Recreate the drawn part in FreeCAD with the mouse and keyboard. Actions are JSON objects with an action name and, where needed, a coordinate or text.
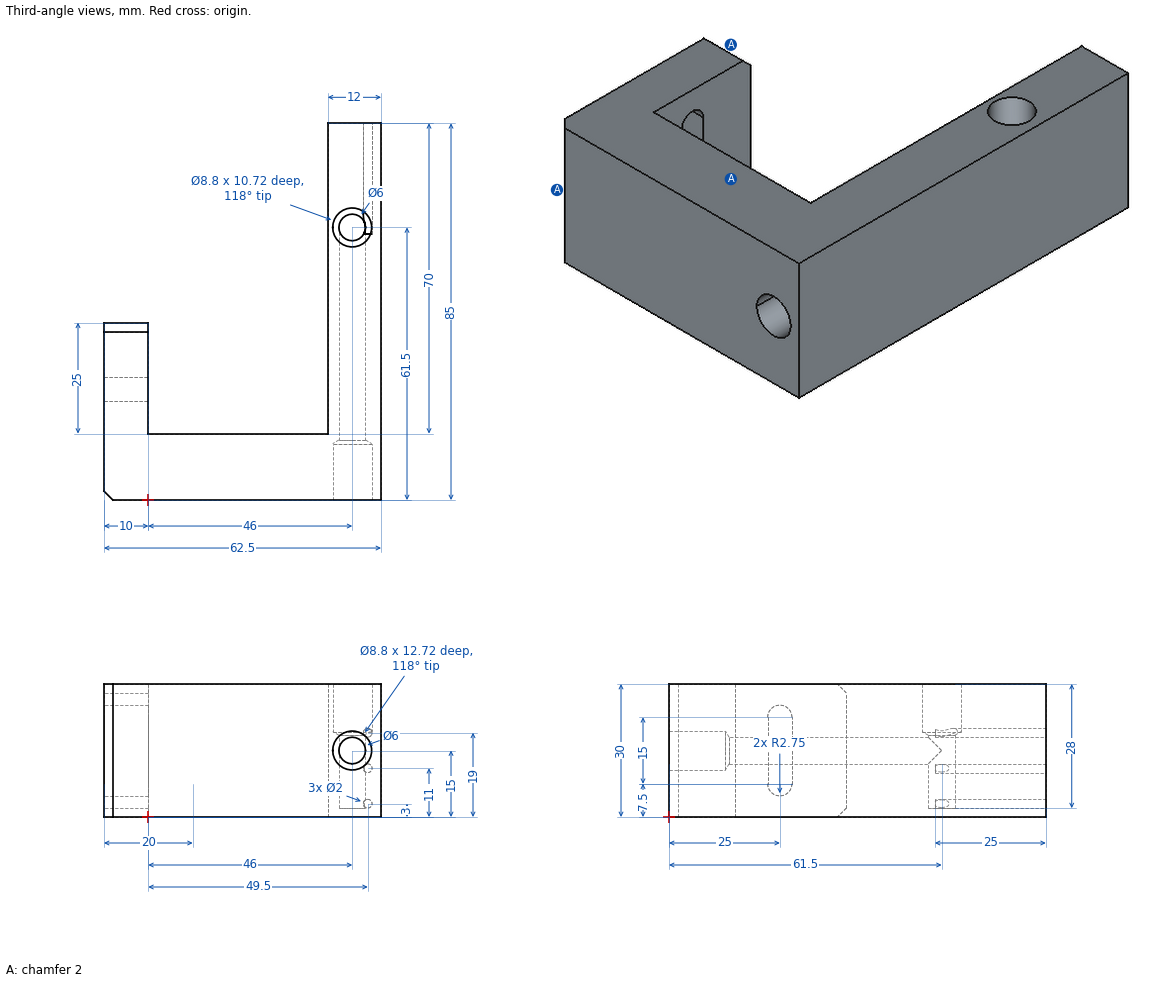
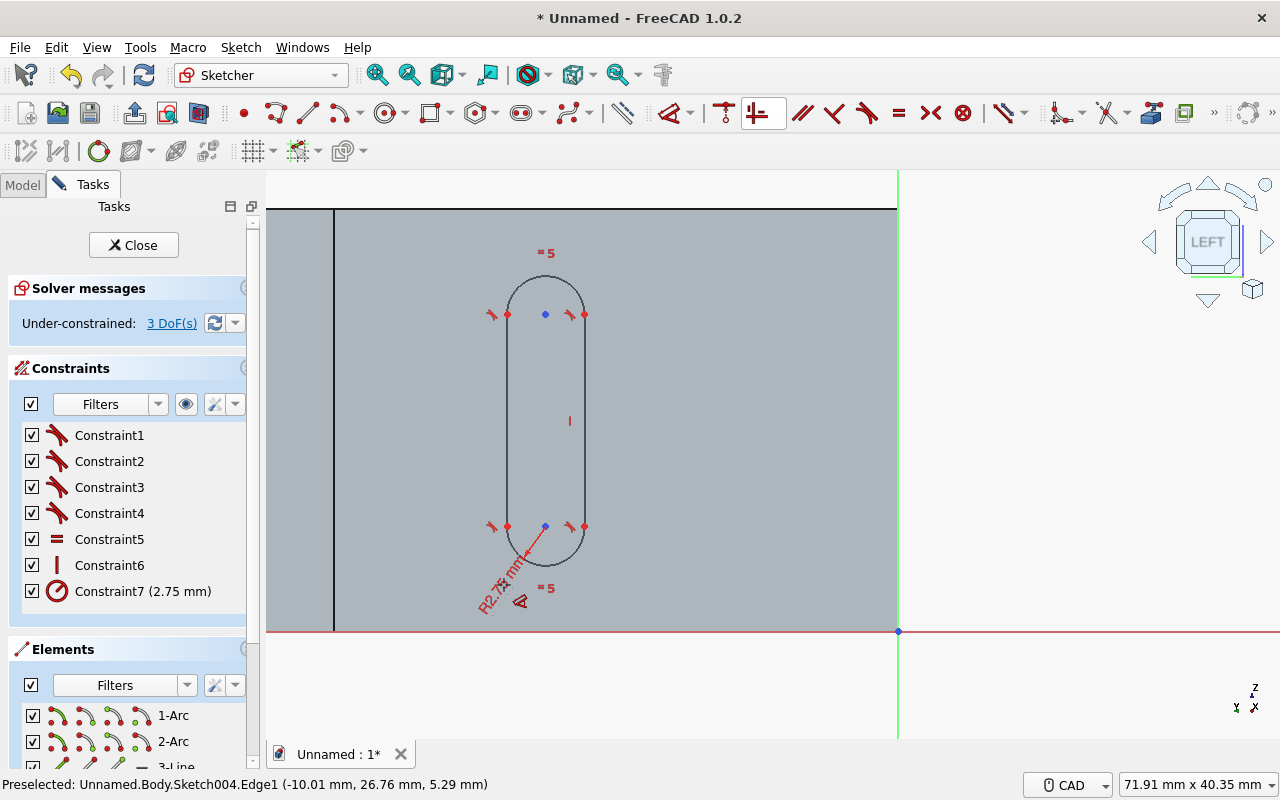
{"action": "left_click", "coordinate": [507, 463]}
{"action": "left_click", "coordinate": [473, 421]}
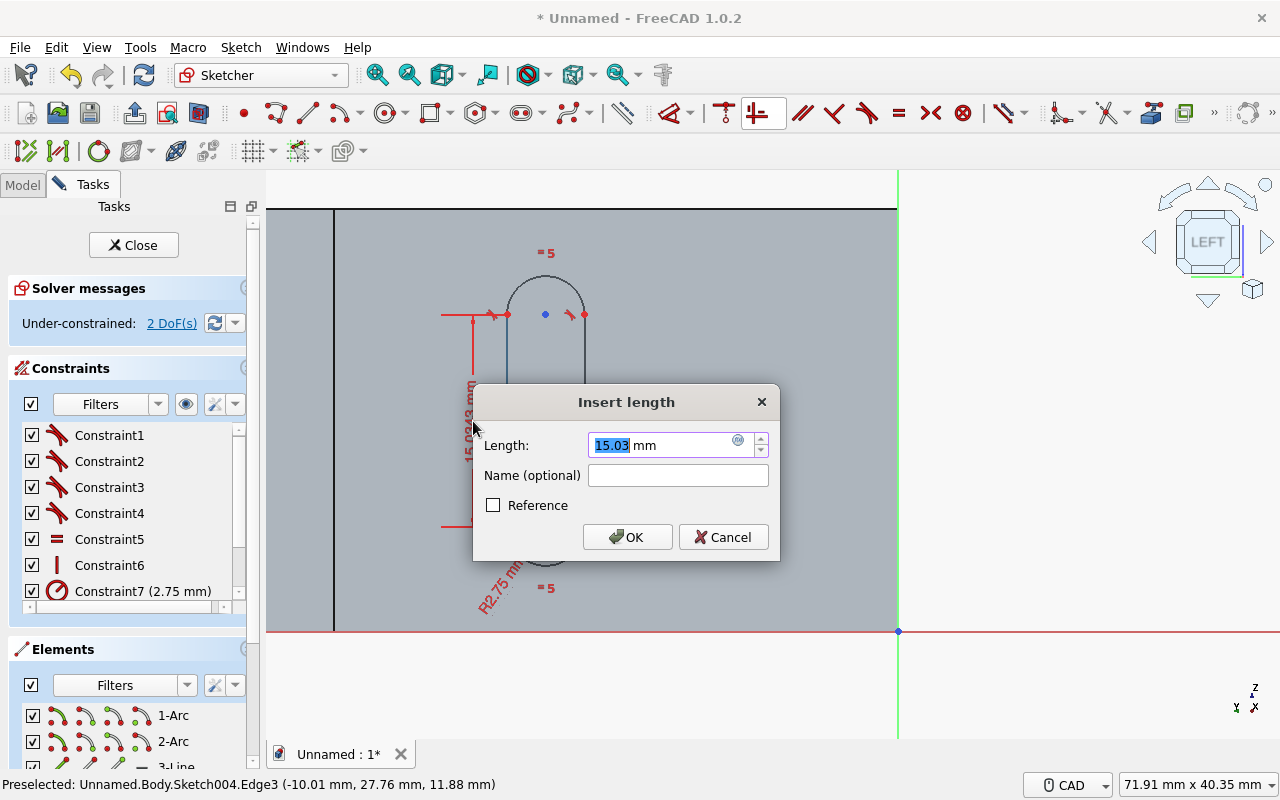
{"action": "type", "text": "15"}
{"action": "key", "text": "Return"}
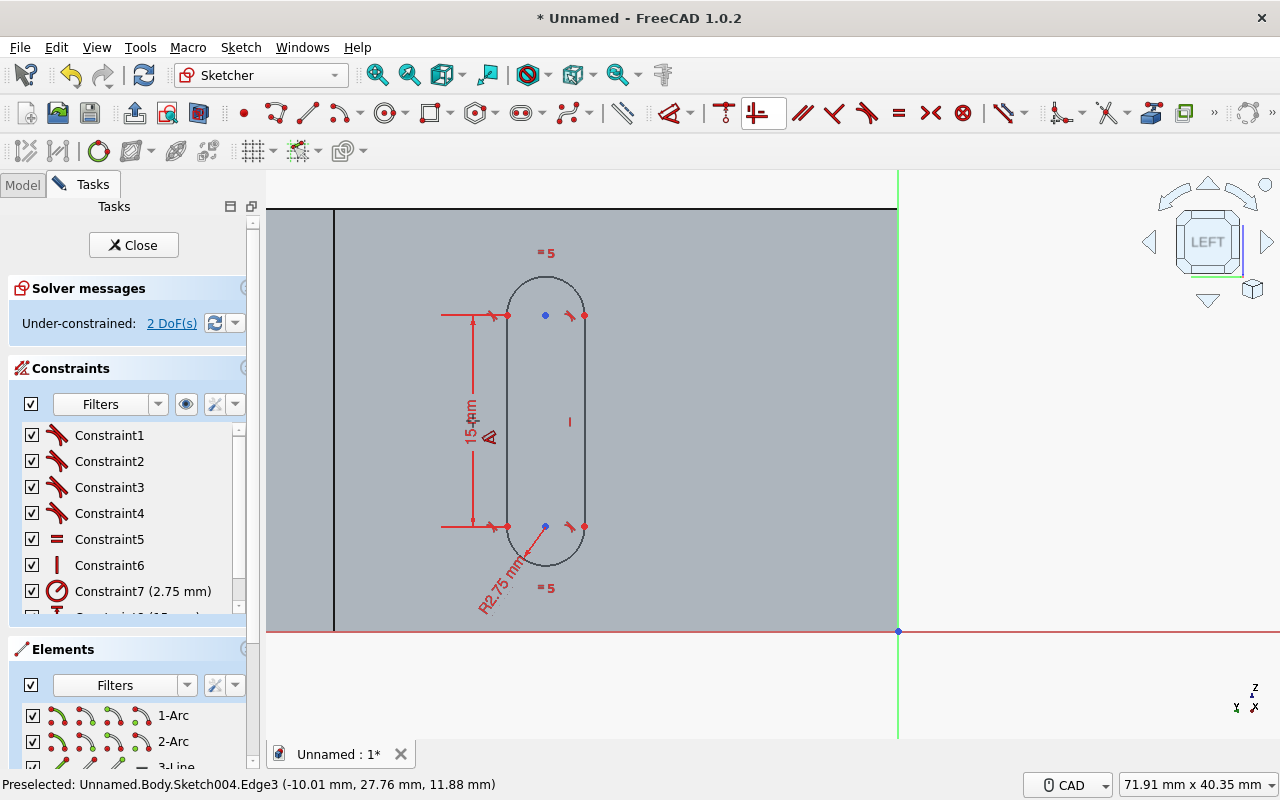
{"action": "left_click", "coordinate": [546, 527]}
{"action": "left_click", "coordinate": [722, 666]}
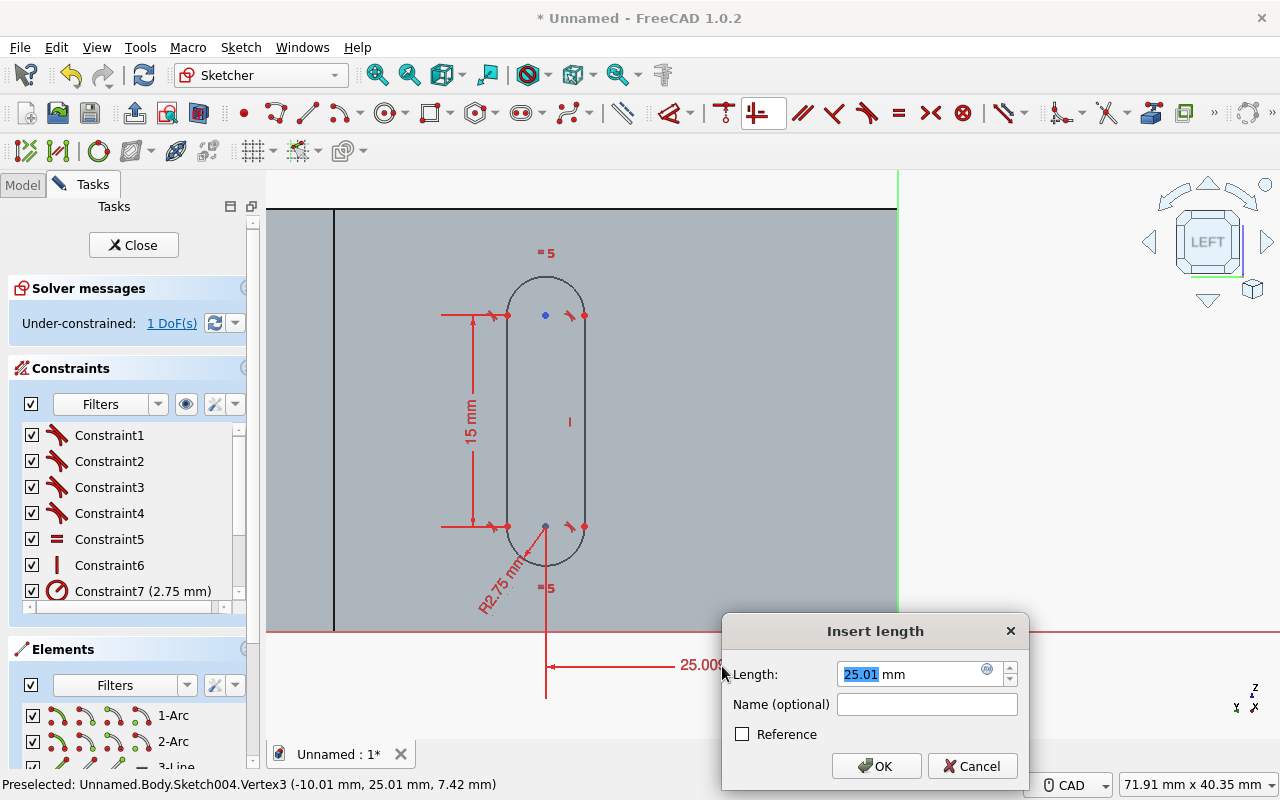
{"action": "type", "text": "25"}
{"action": "key", "text": "Return"}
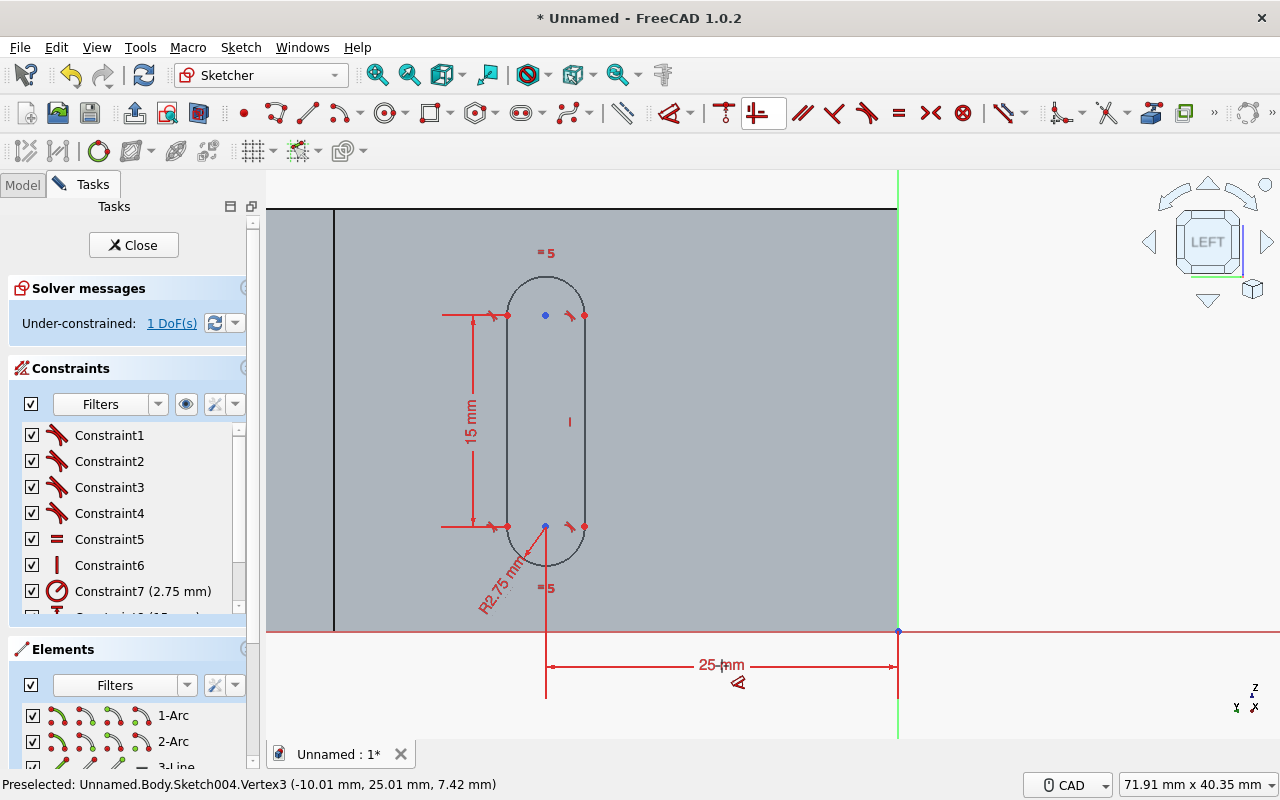
{"action": "left_click", "coordinate": [507, 527]}
{"action": "left_click", "coordinate": [932, 579]}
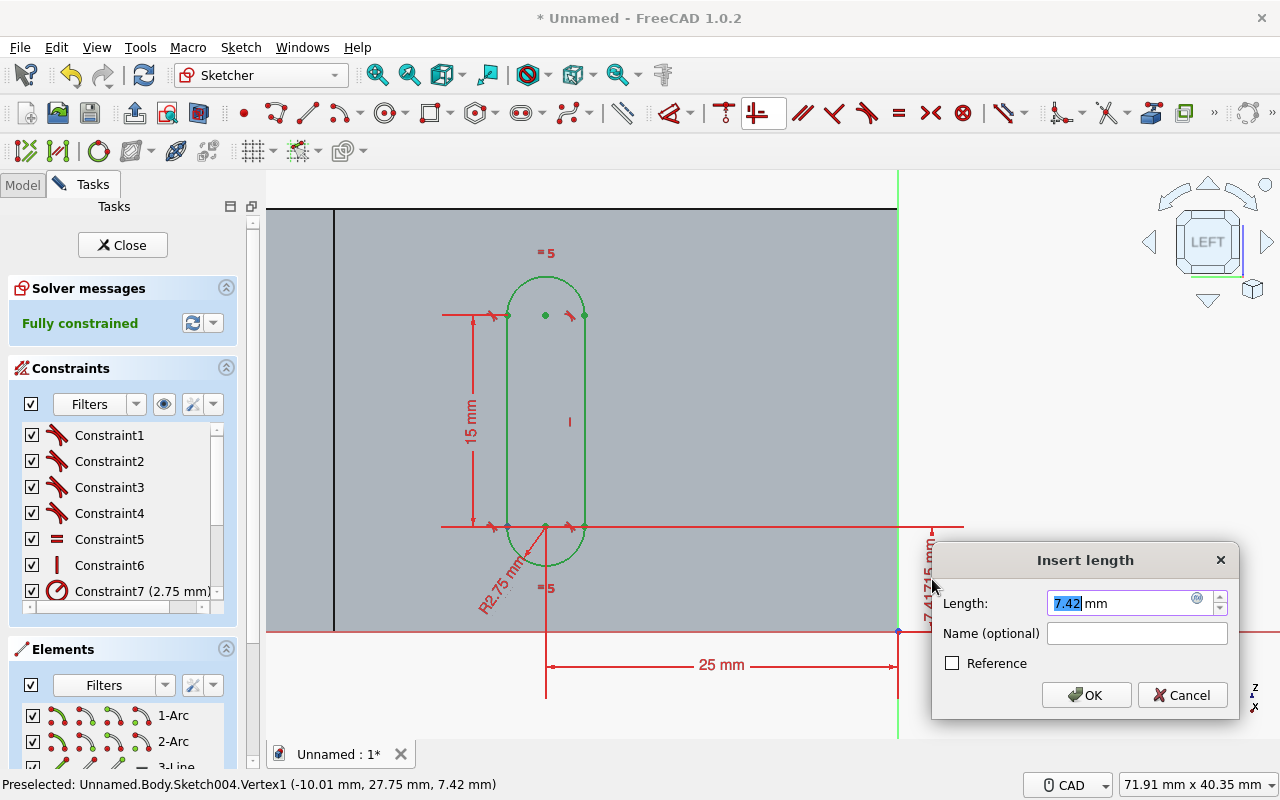
{"action": "type", "text": "7.5"}
{"action": "key", "text": "Return"}
{"action": "key", "text": "Escape"}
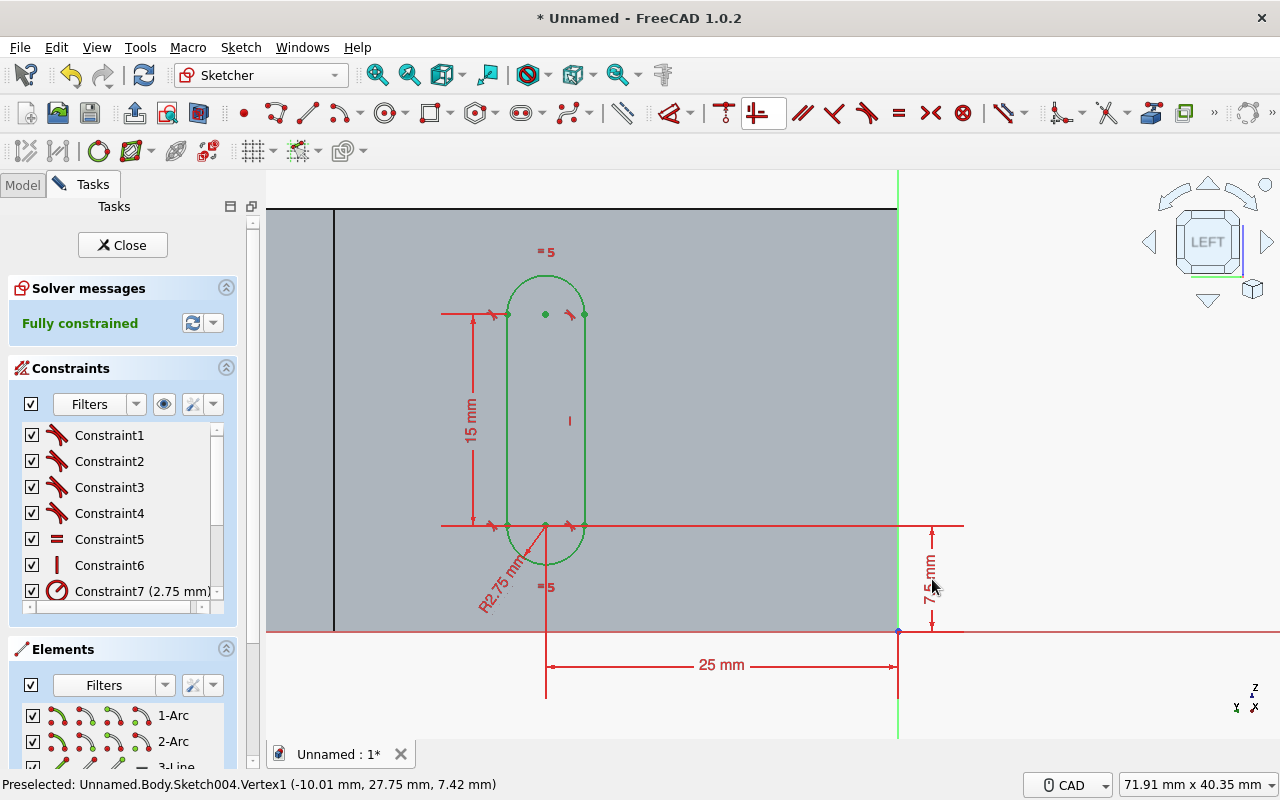
{"action": "left_click", "coordinate": [123, 245]}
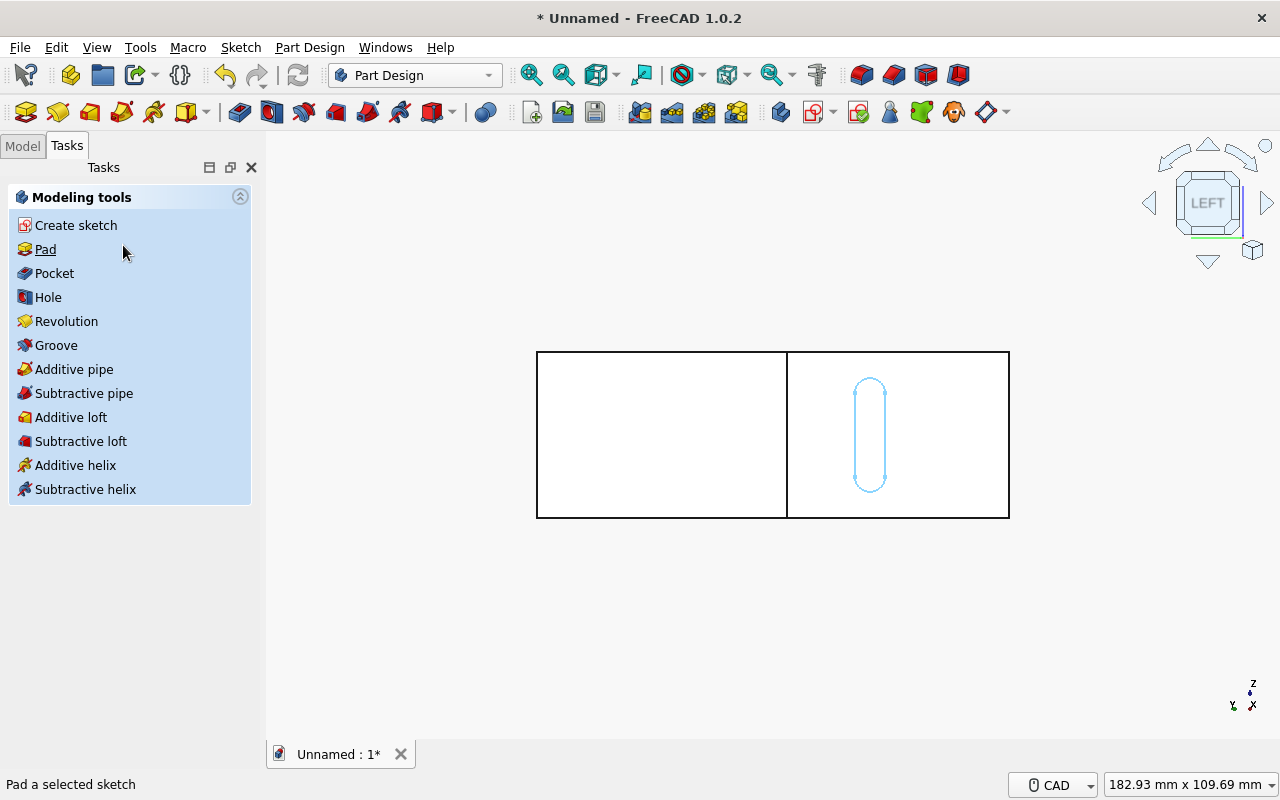
{"action": "left_click", "coordinate": [240, 112]}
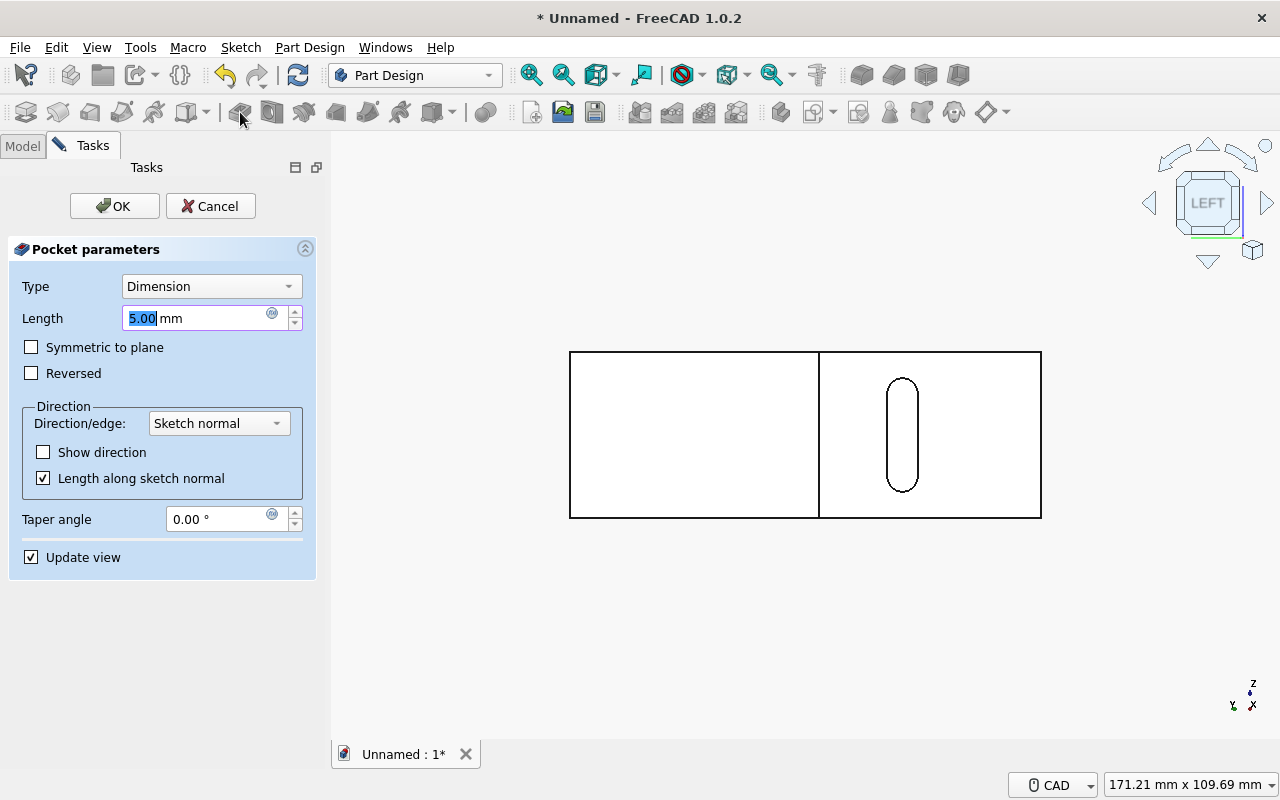
{"action": "type", "text": "20"}
{"action": "key", "text": "Tab"}